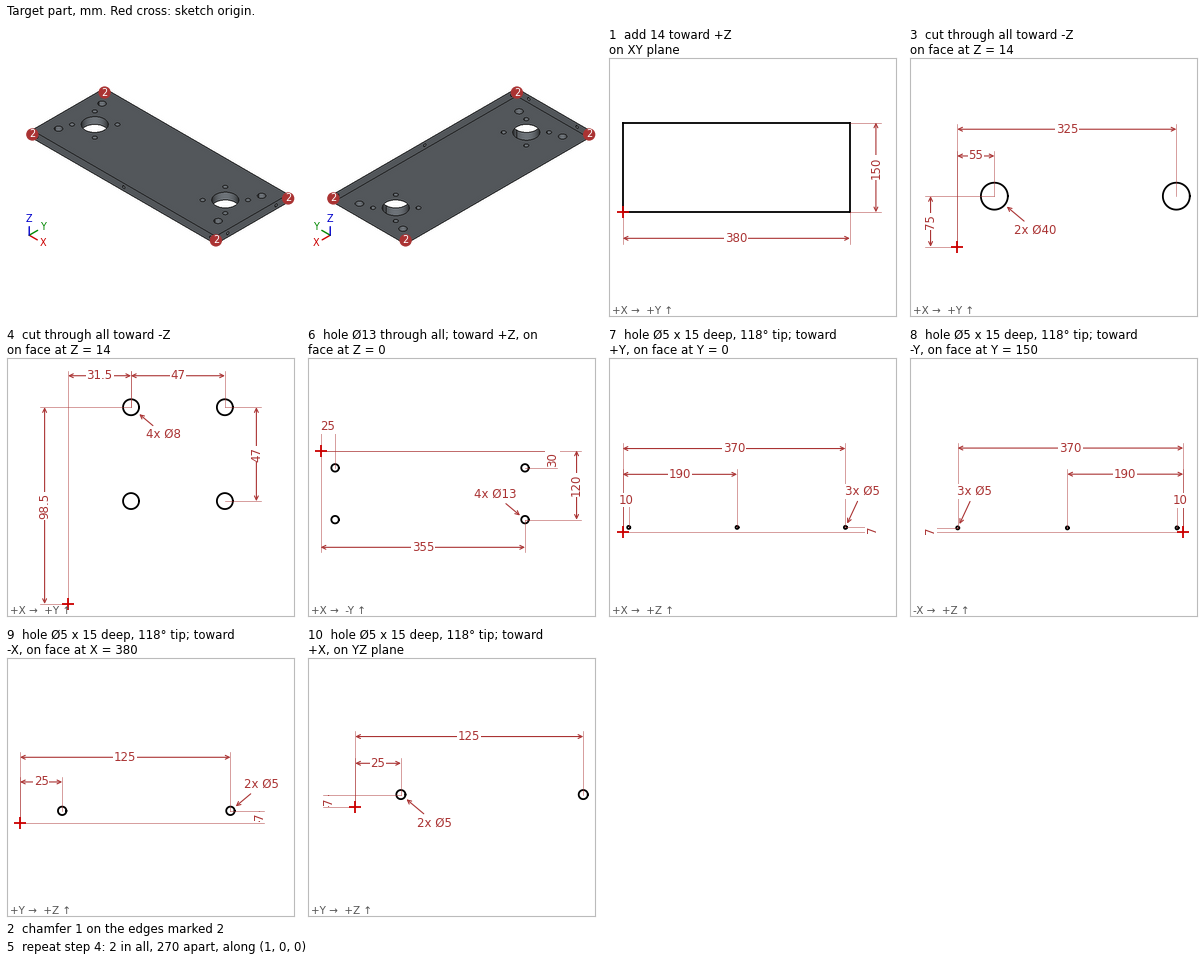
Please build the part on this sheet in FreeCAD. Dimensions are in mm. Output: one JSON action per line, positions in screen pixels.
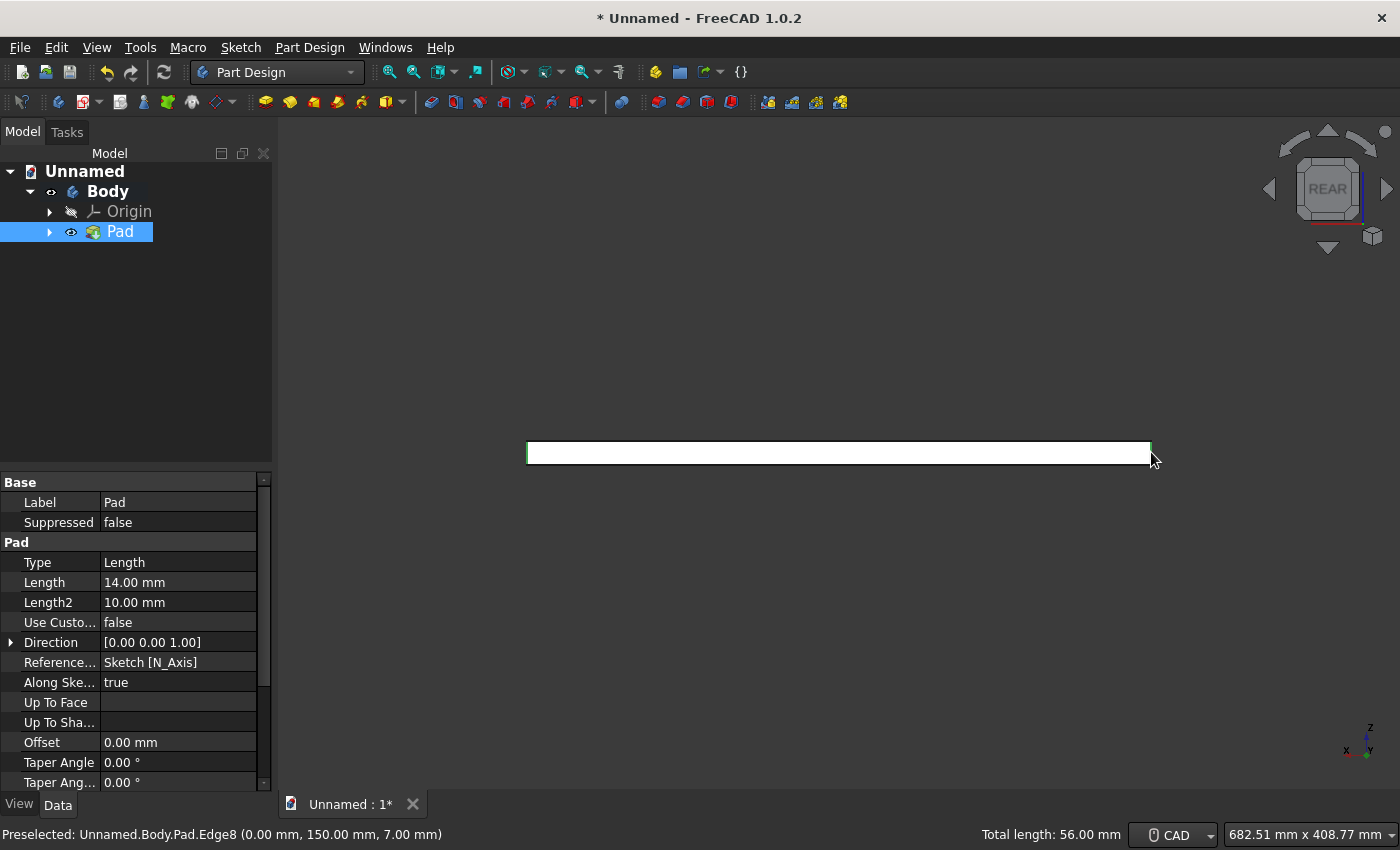
{"action": "left_click", "coordinate": [684, 102]}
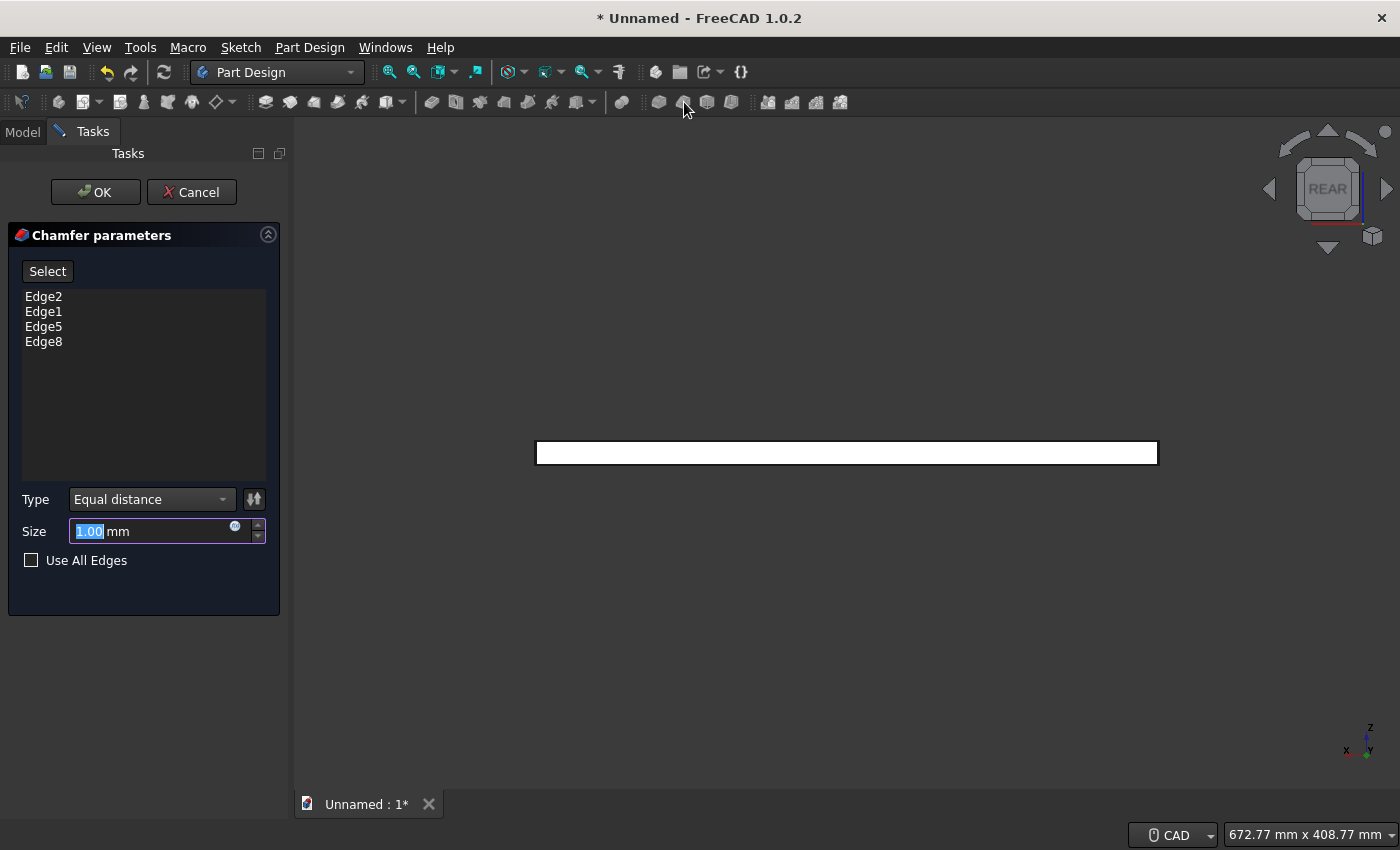
{"action": "type", "text": "1"}
{"action": "key", "text": "Tab"}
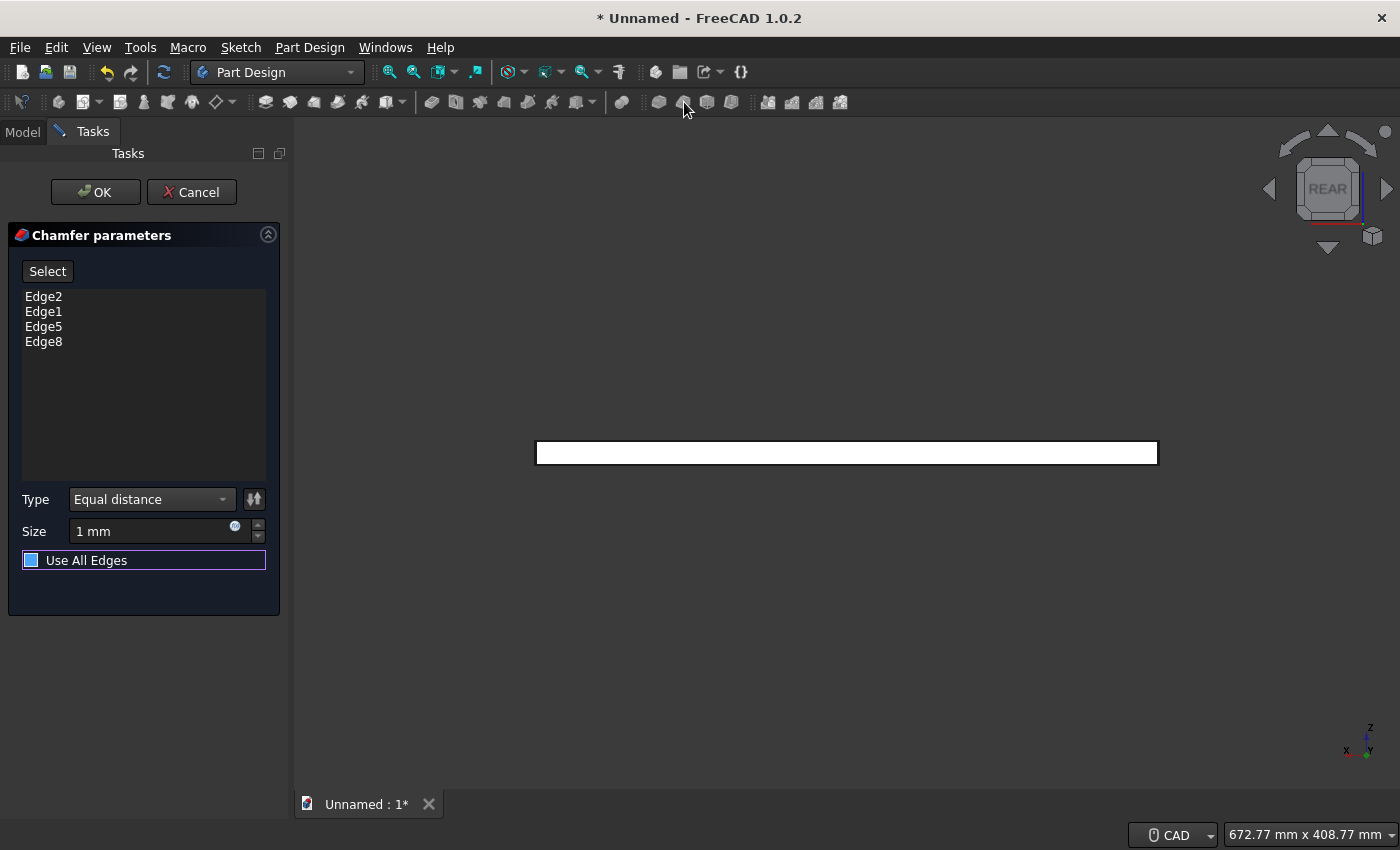
{"action": "left_click", "coordinate": [96, 192]}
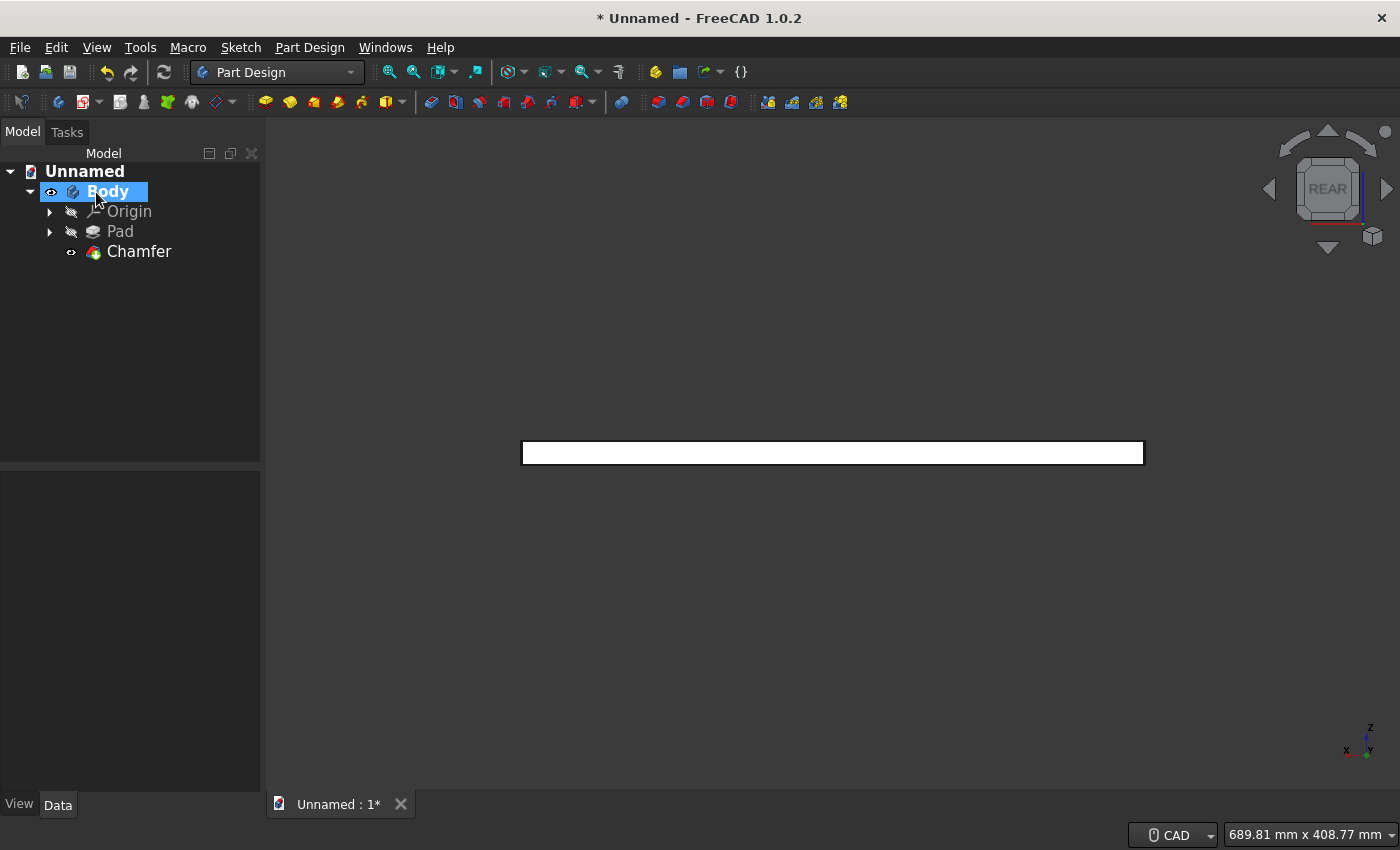
{"action": "key", "text": "0"}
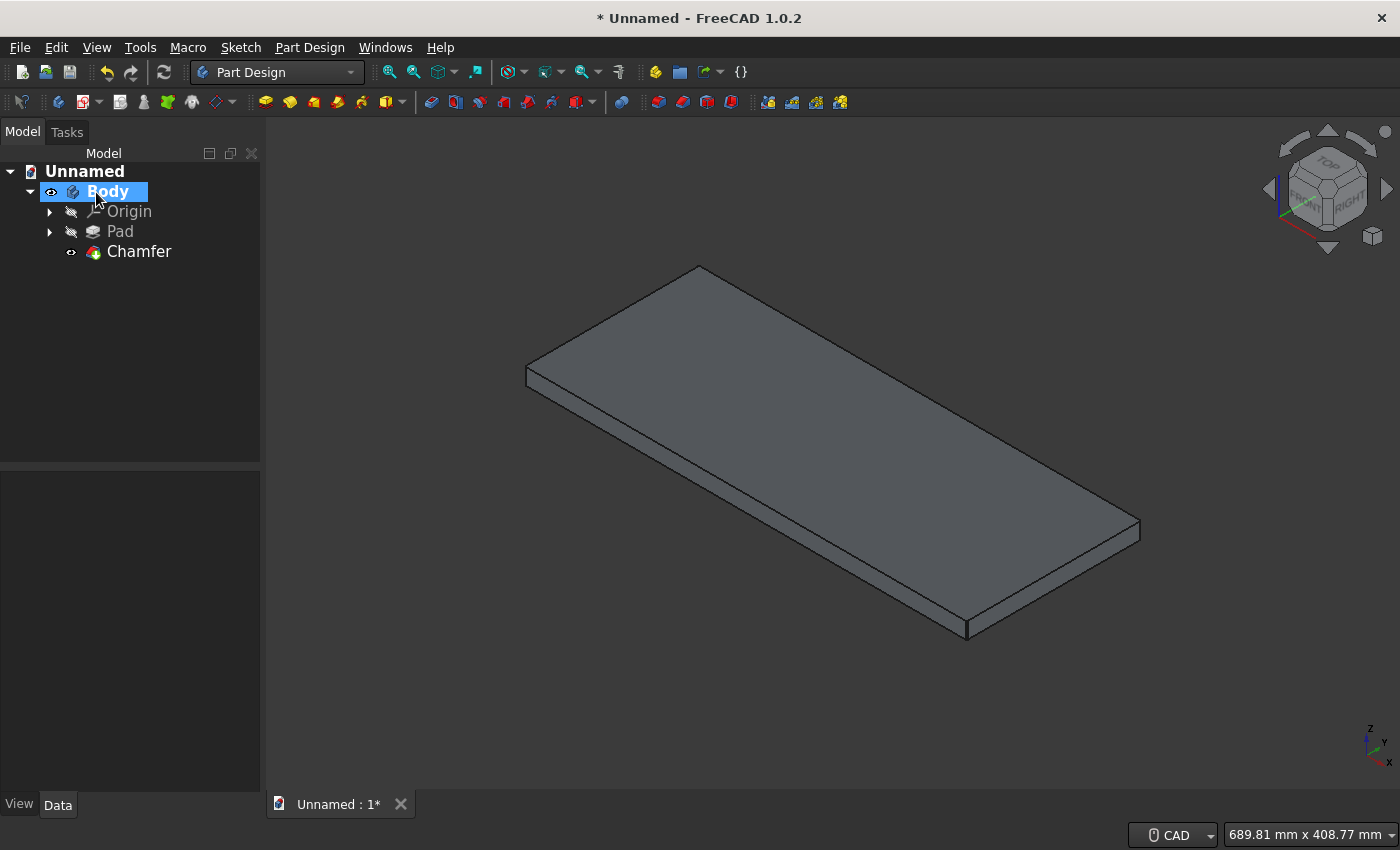
{"action": "left_click", "coordinate": [959, 515]}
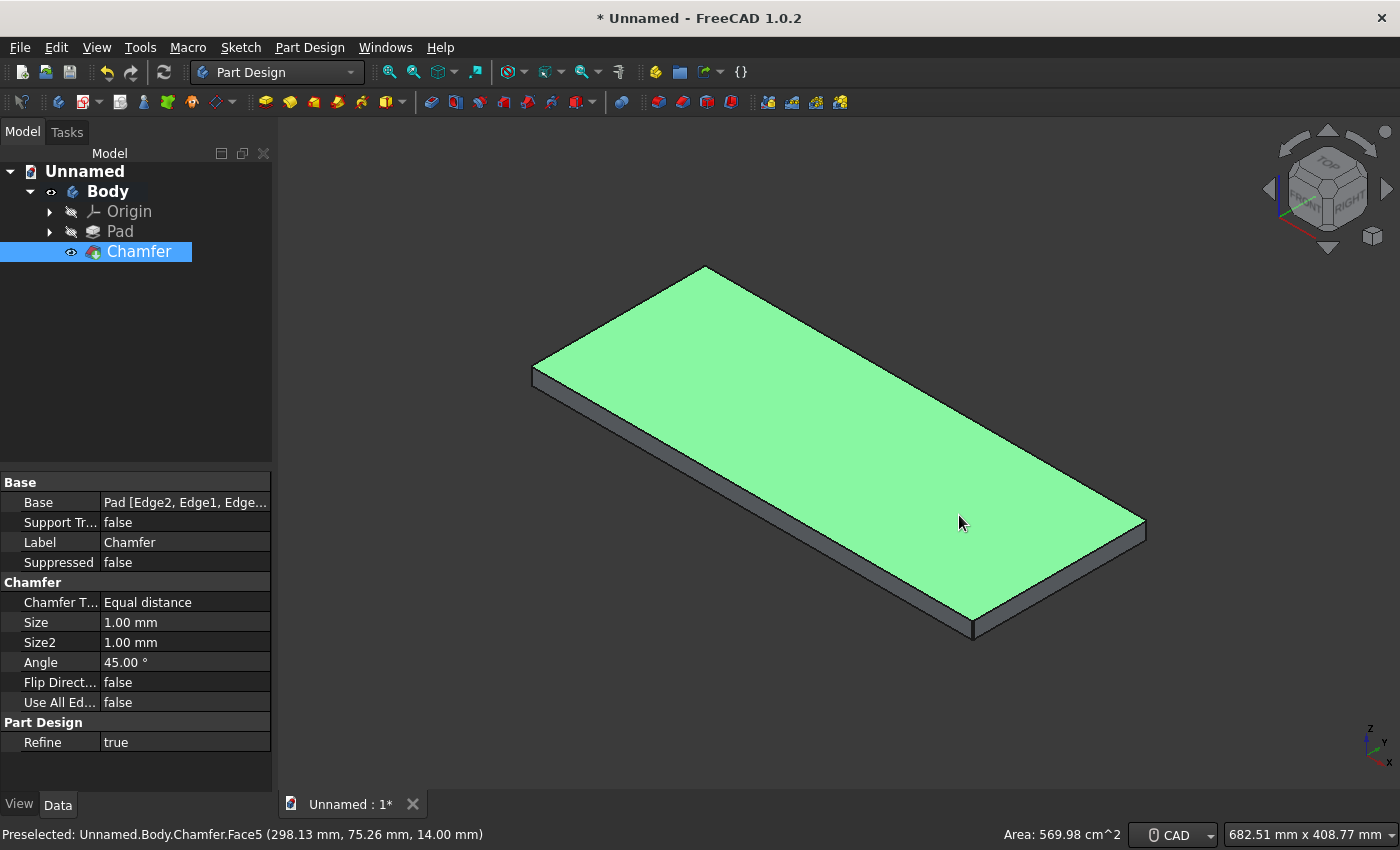
{"action": "left_click", "coordinate": [84, 102]}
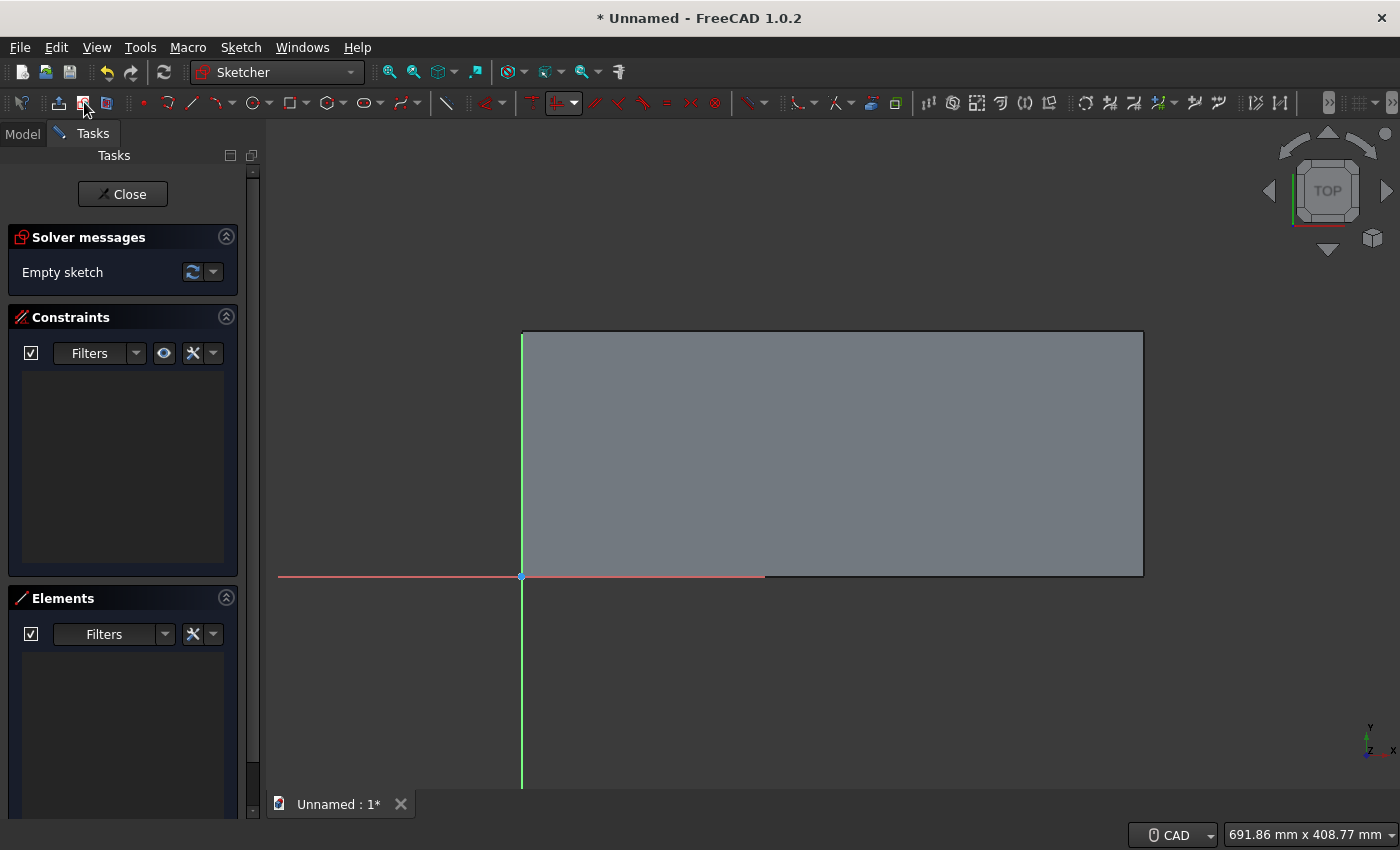
{"action": "left_click", "coordinate": [254, 104]}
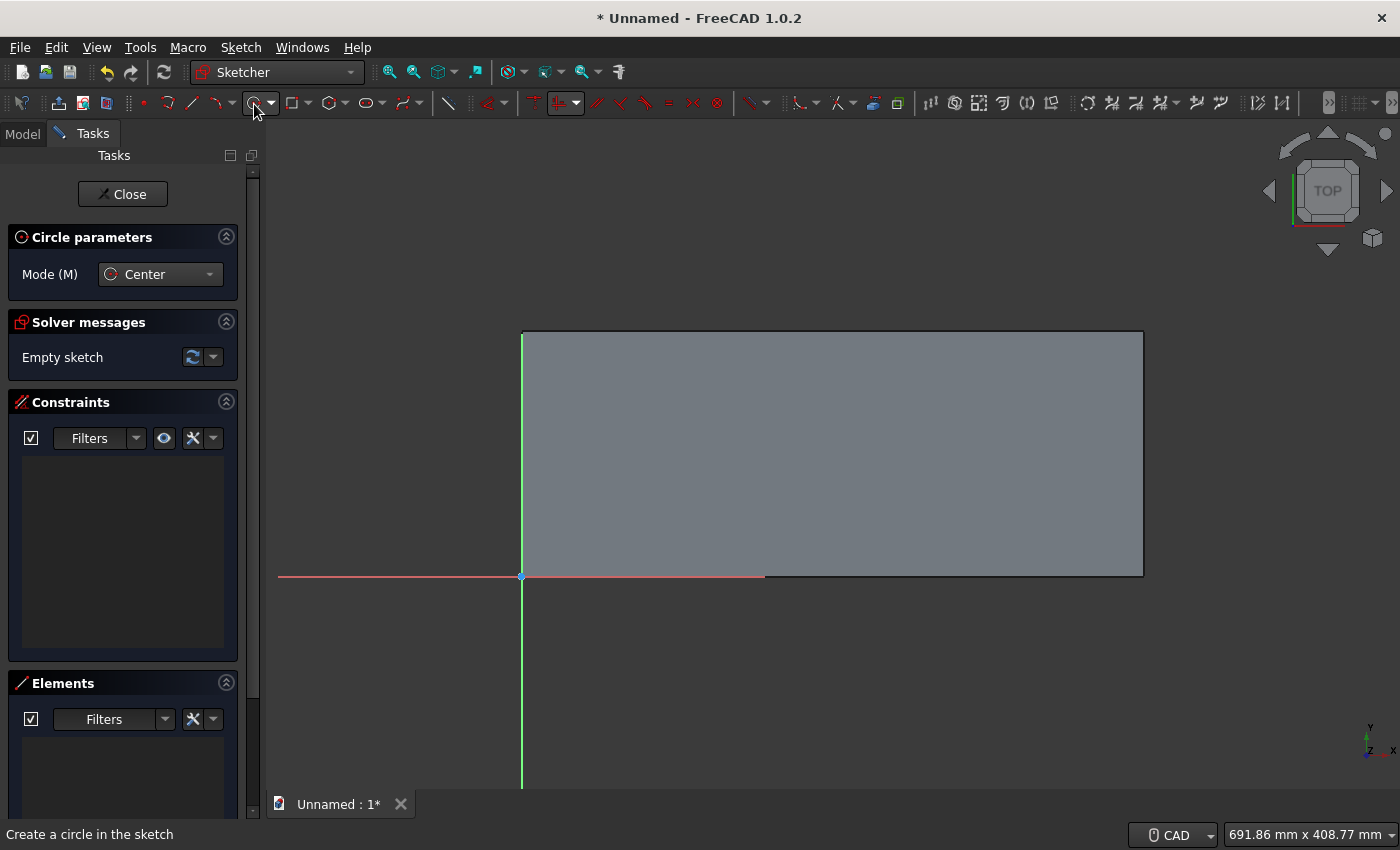
{"action": "left_click", "coordinate": [612, 454]}
{"action": "mouse_move", "coordinate": [635, 431]}